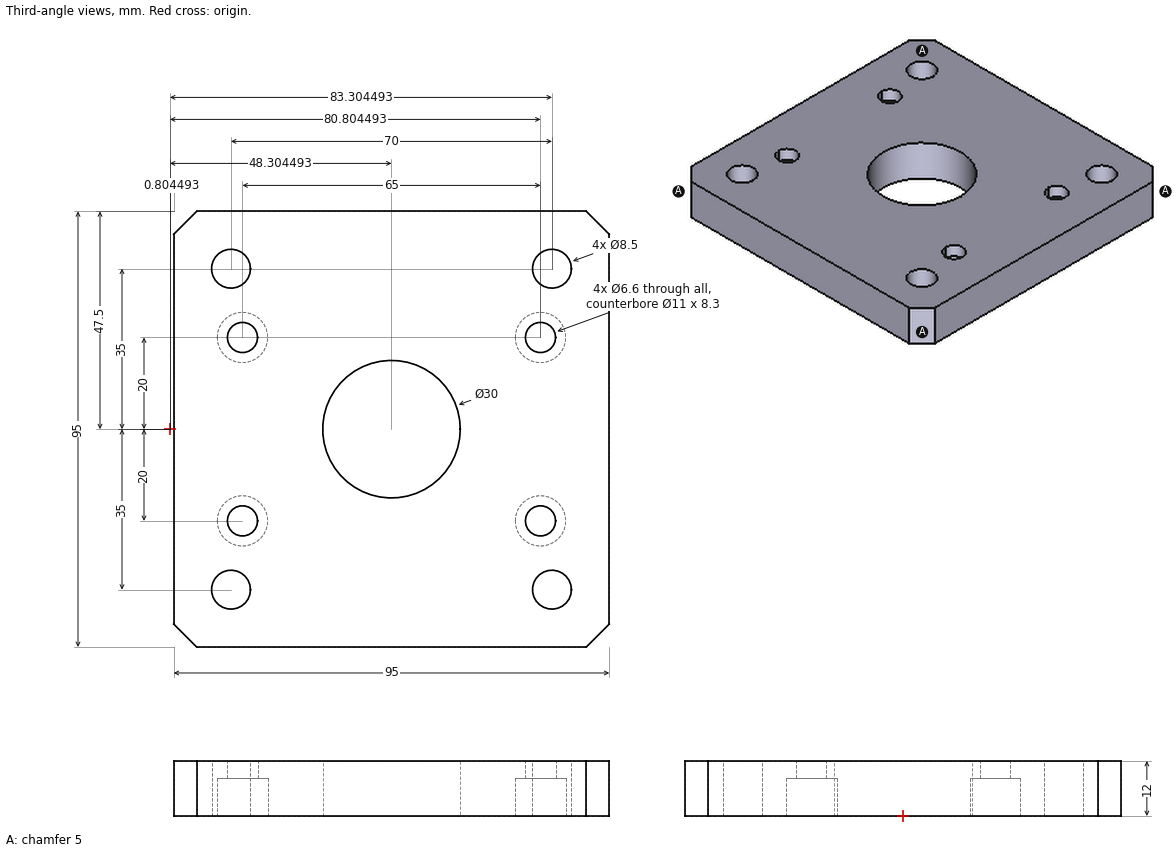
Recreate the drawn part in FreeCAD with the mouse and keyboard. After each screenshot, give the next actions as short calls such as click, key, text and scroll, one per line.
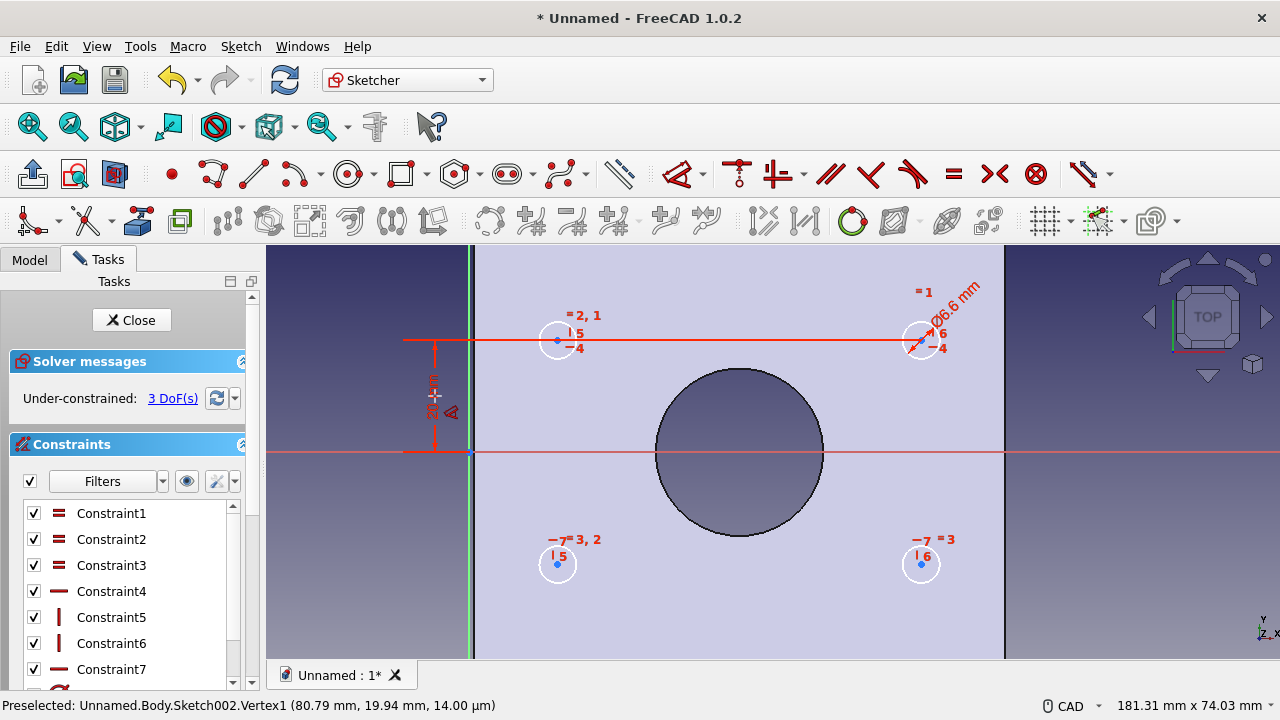
click(558, 565)
click(435, 508)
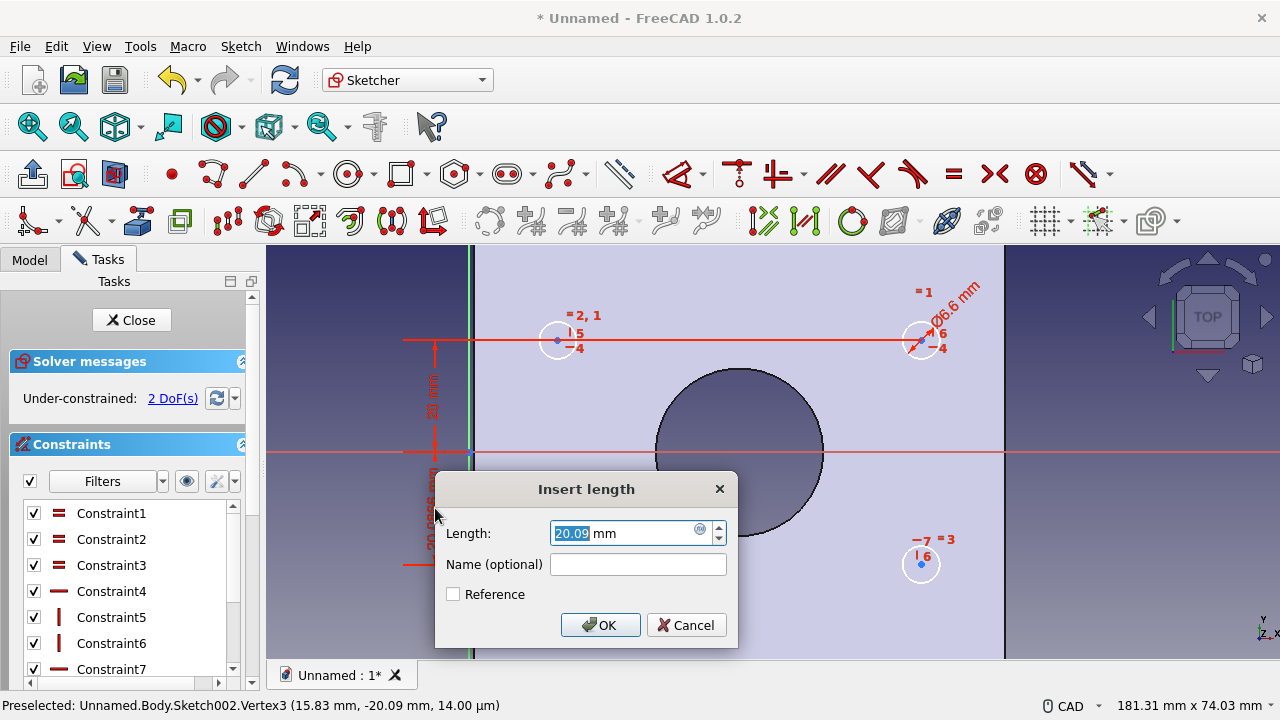
text(20)
key(Return)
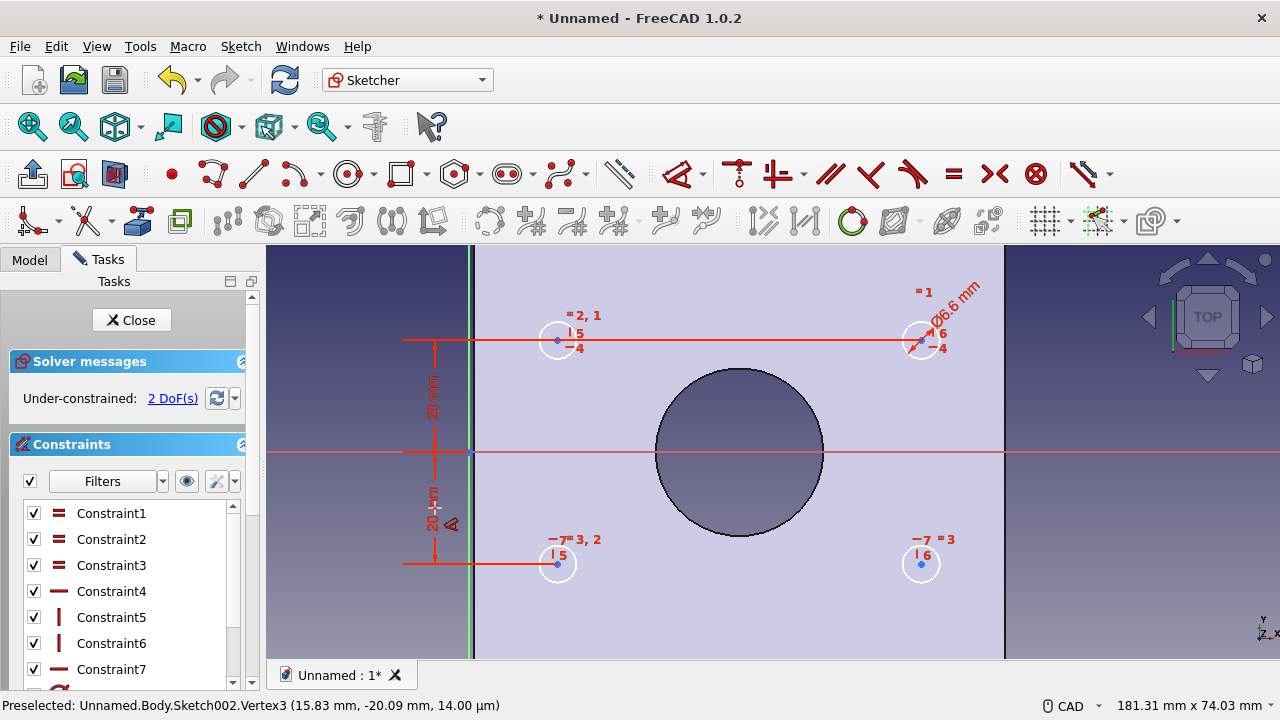
click(921, 340)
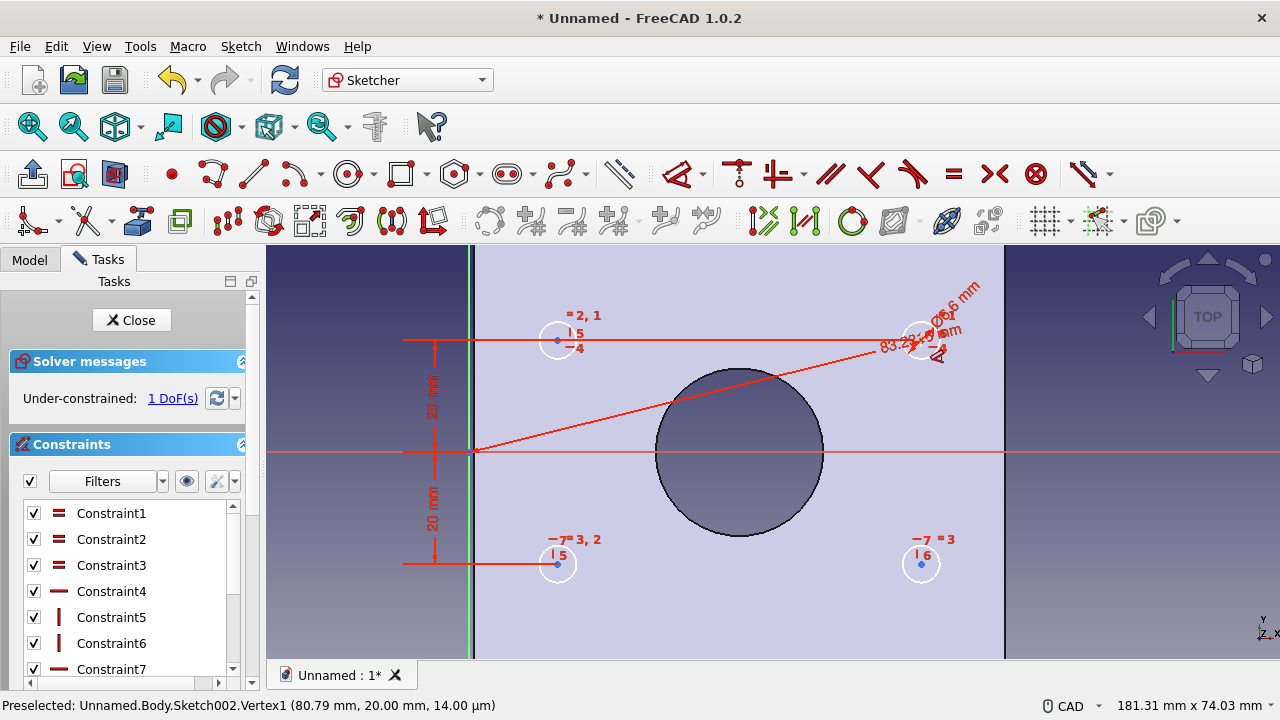
click(558, 340)
click(740, 306)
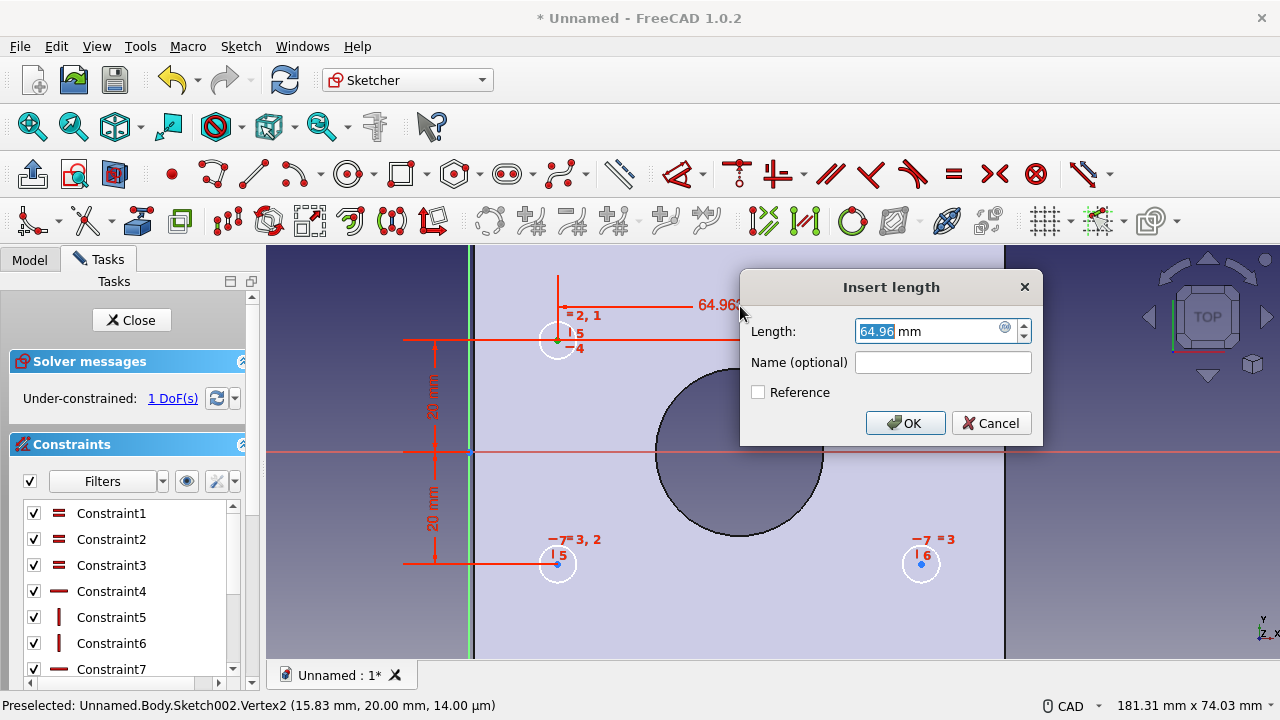
text(65)
key(Return)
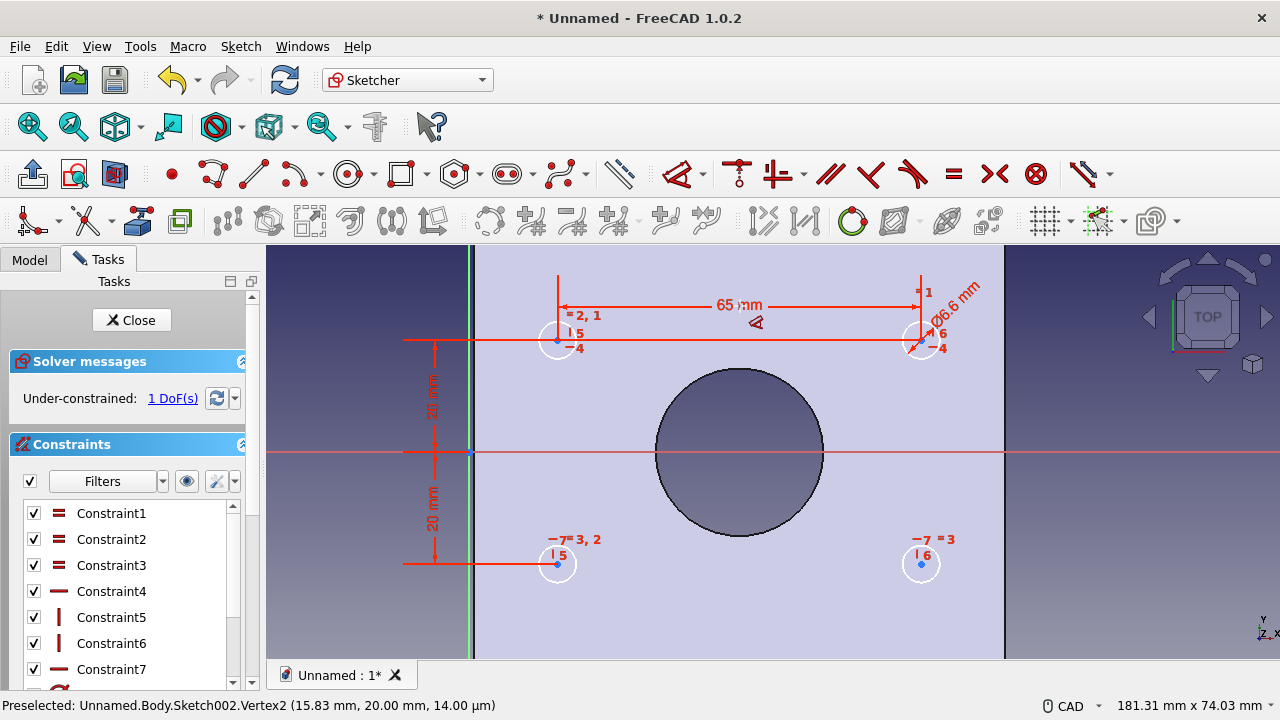
click(921, 340)
click(591, 306)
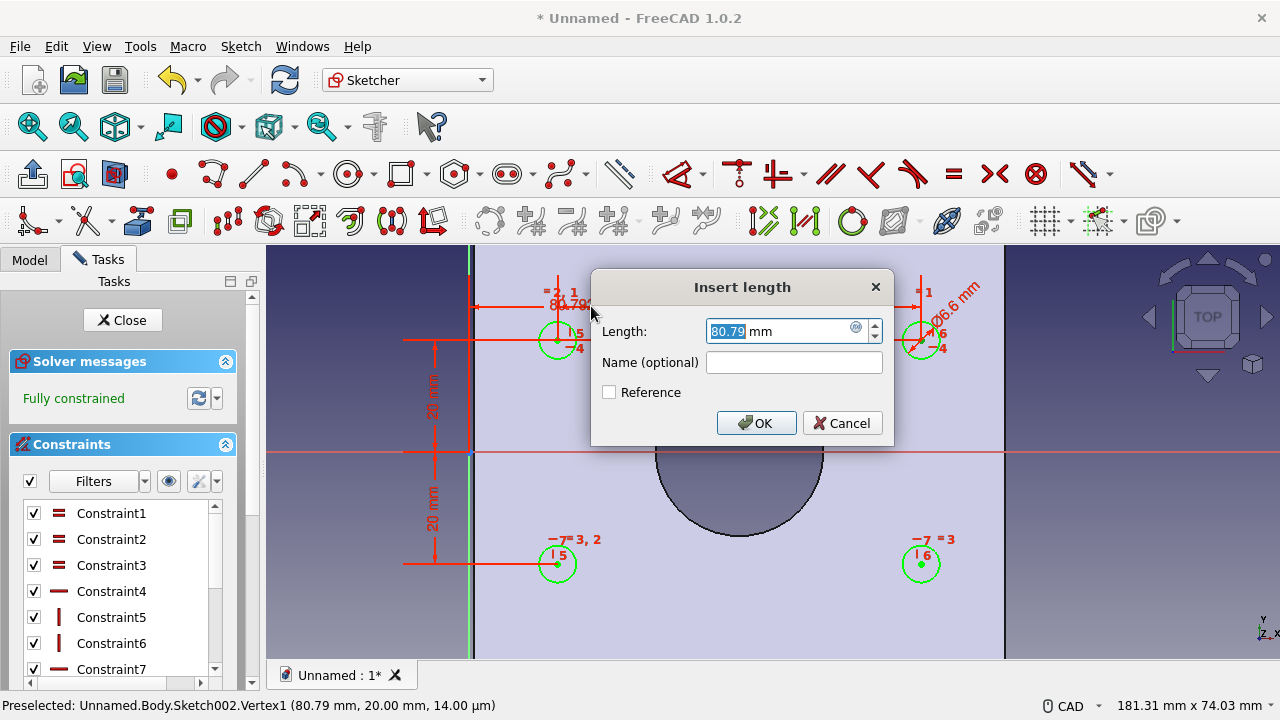
text(80.804493)
key(Return)
key(Escape)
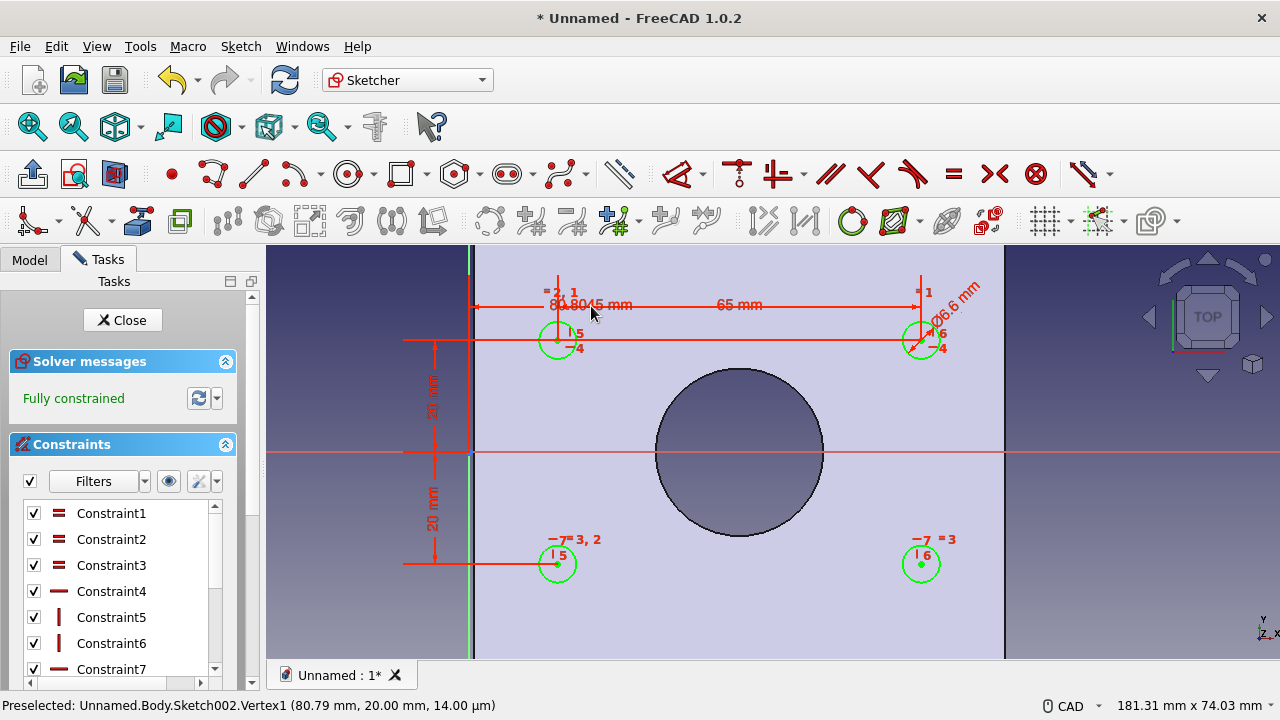
click(123, 320)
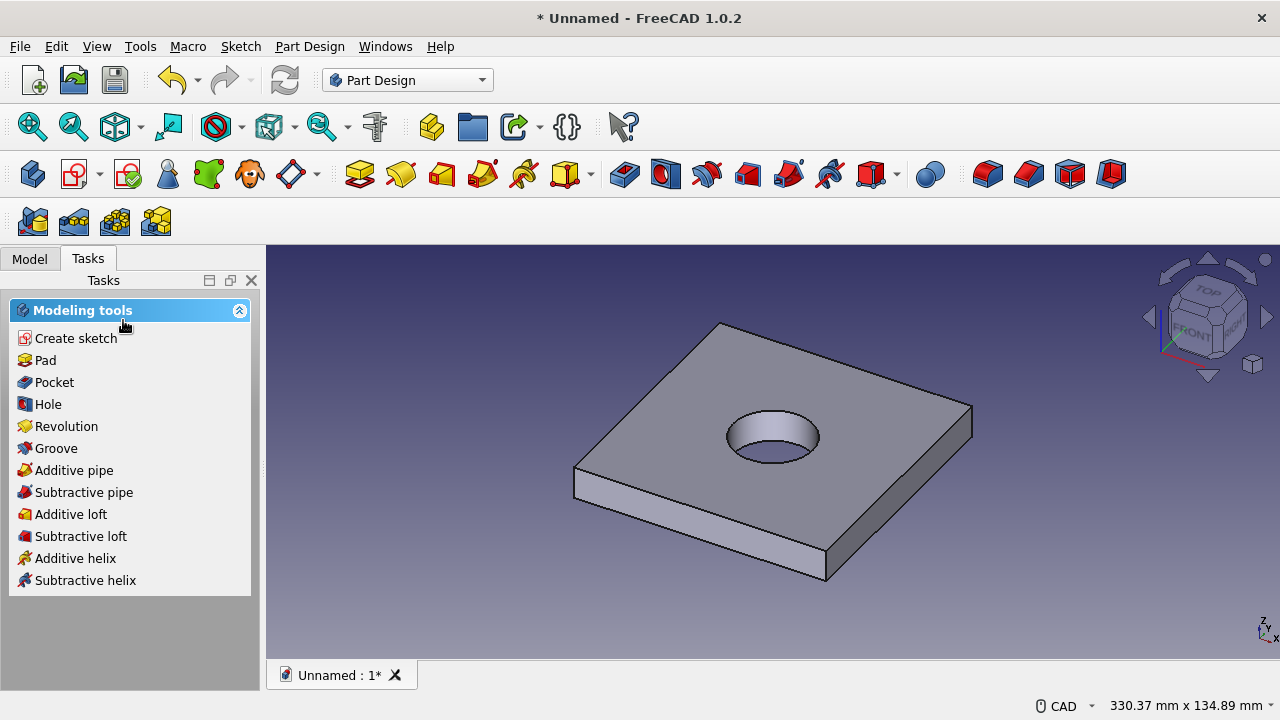
click(666, 174)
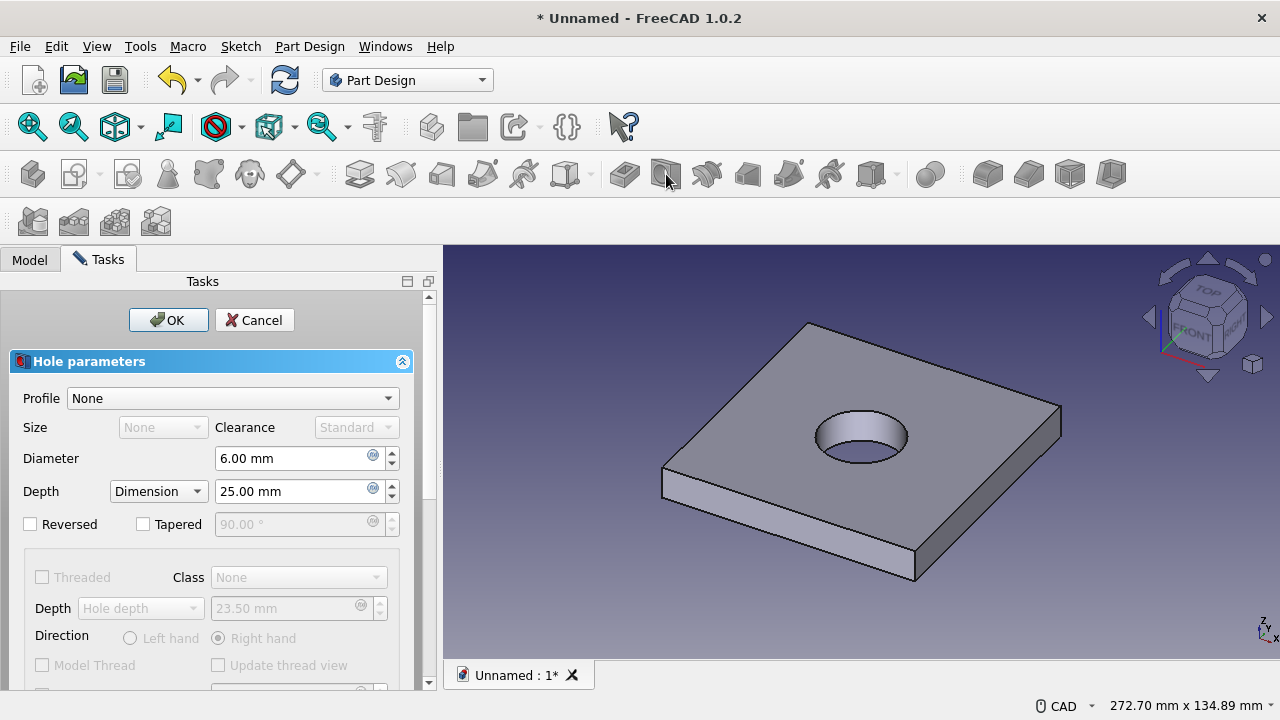
triple_click(300, 458)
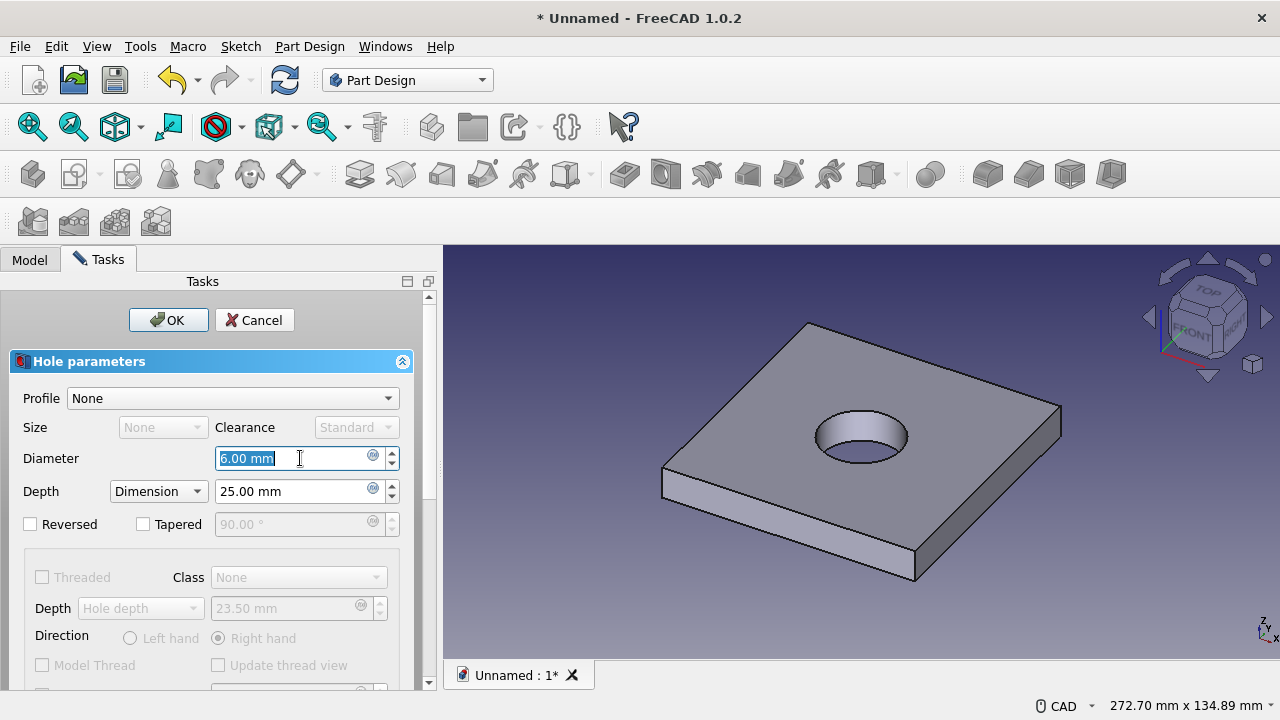
text(6.6)
key(Tab)